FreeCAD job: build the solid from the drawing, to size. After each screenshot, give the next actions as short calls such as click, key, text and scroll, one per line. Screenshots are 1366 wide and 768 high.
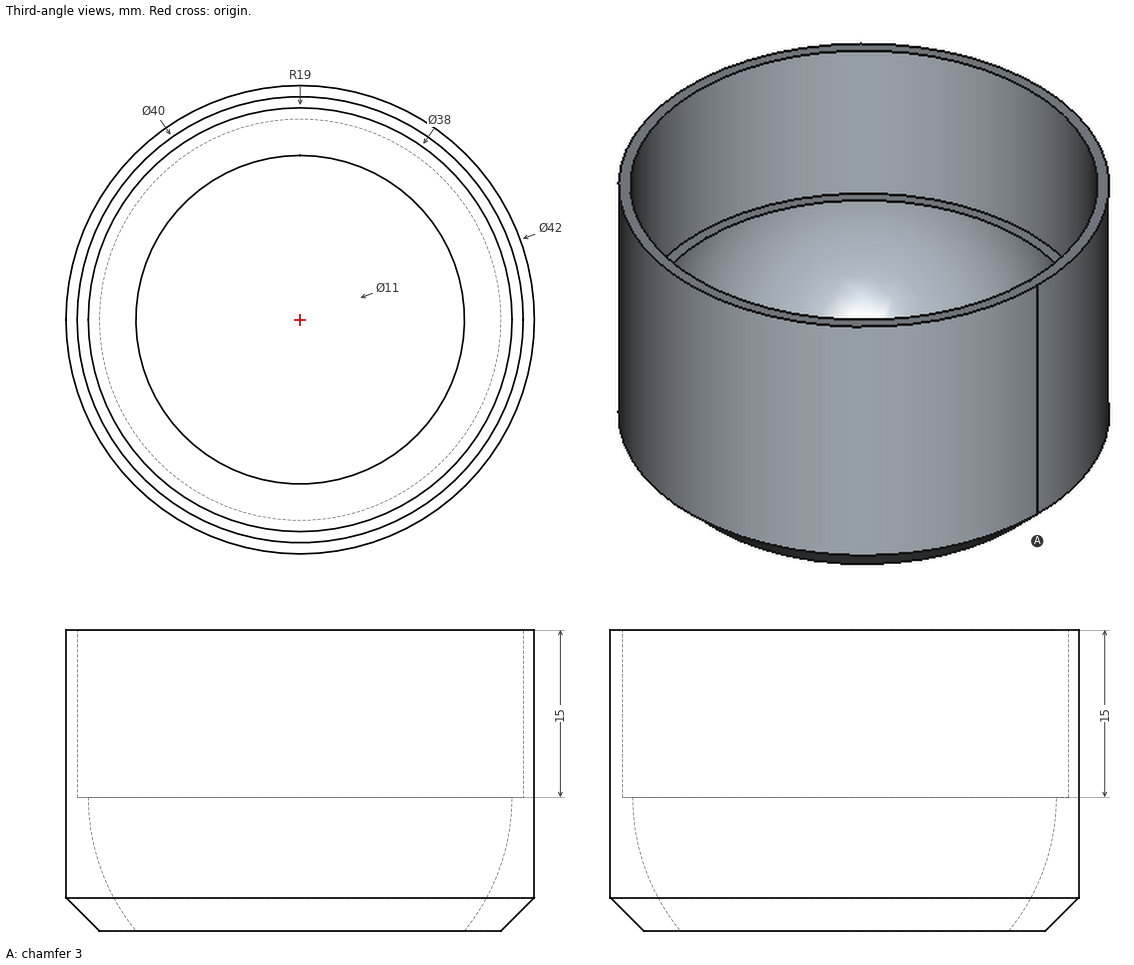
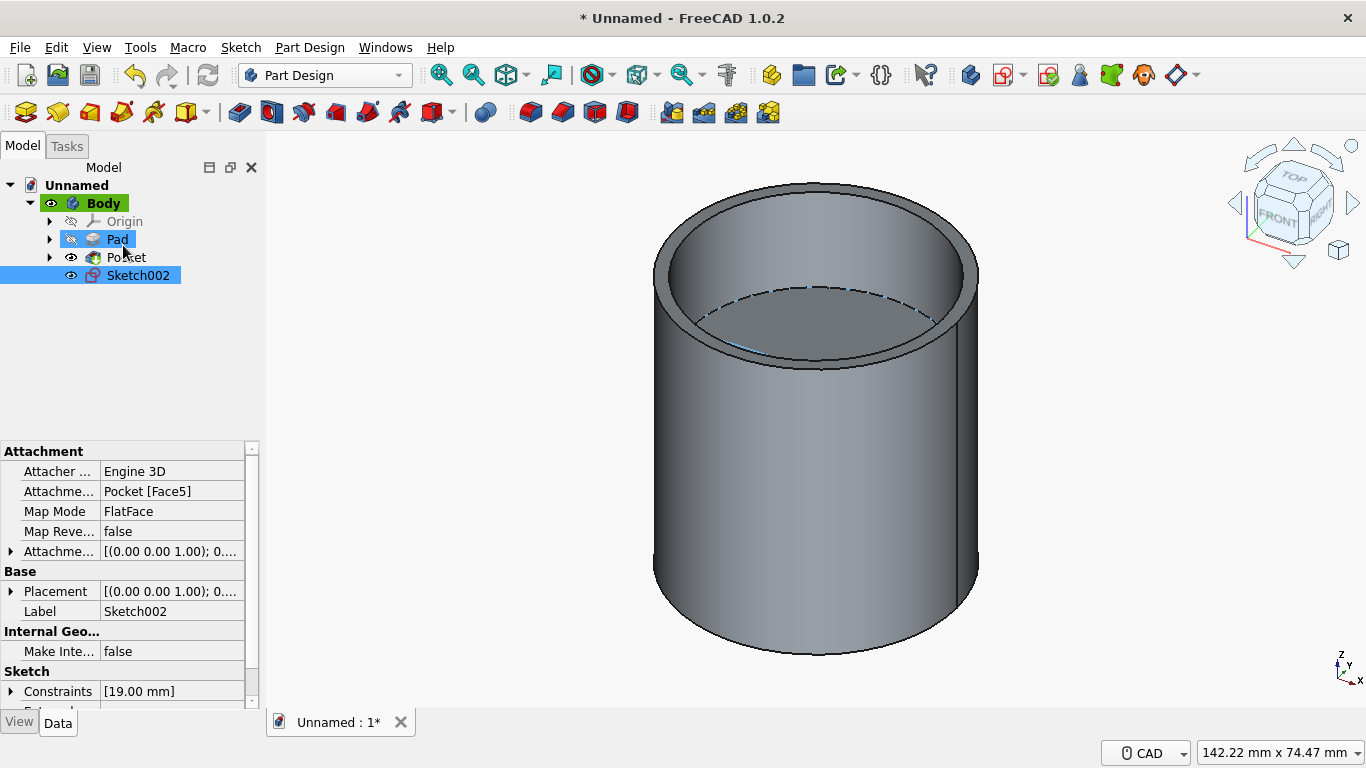
click(304, 112)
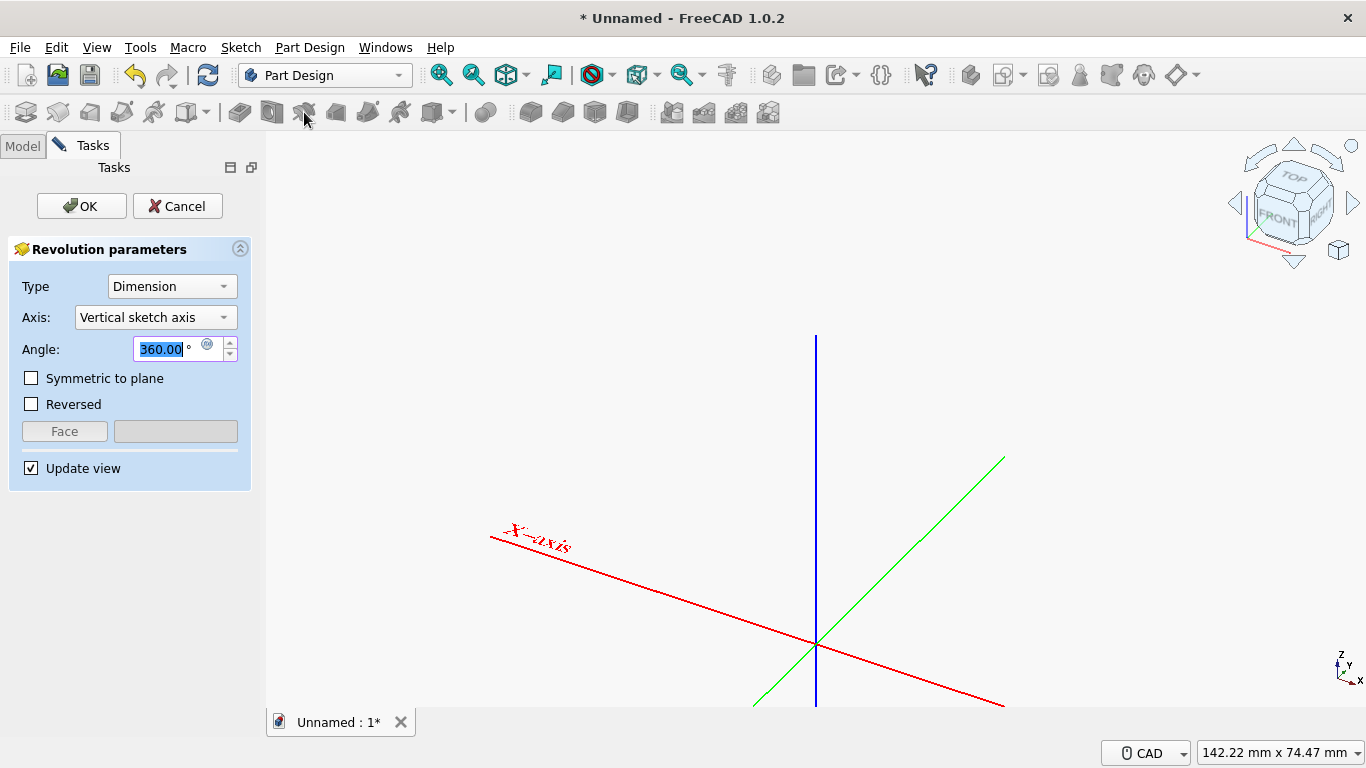
click(156, 318)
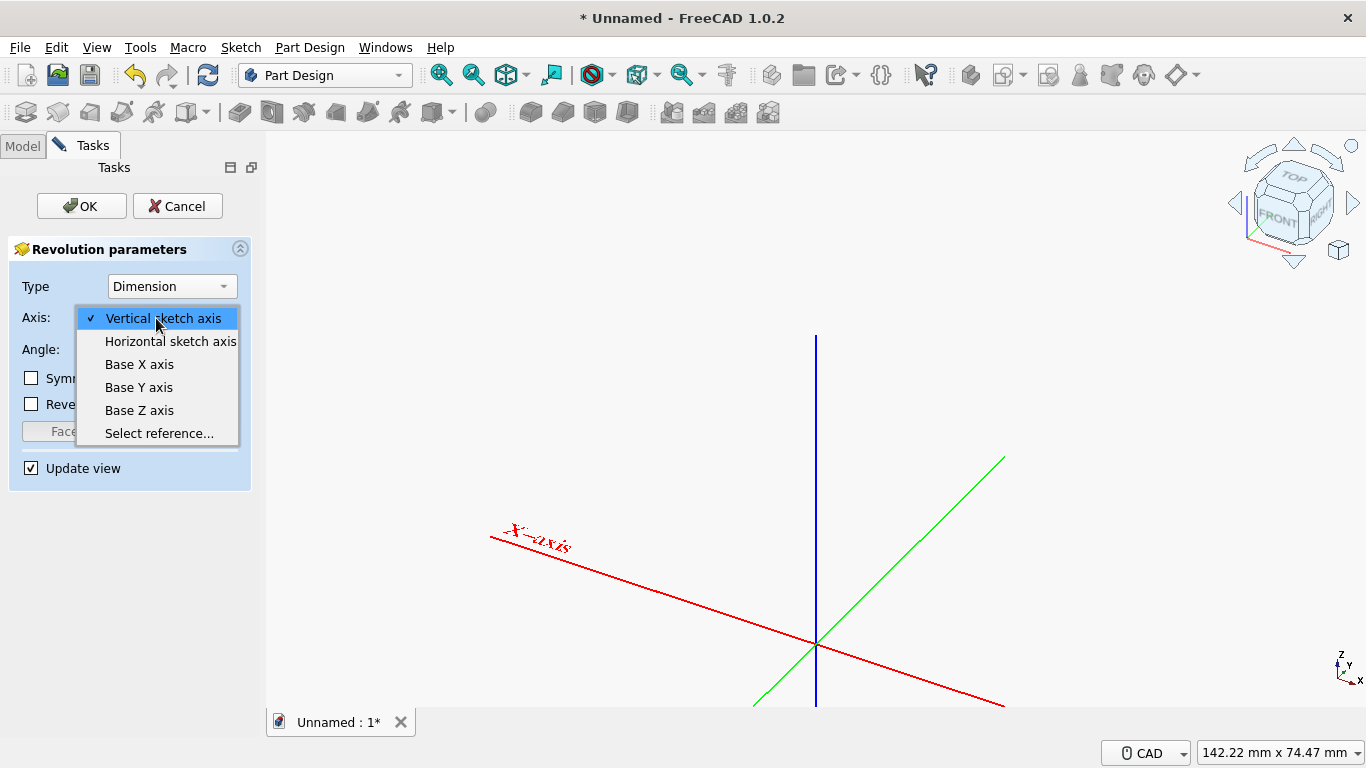
click(156, 342)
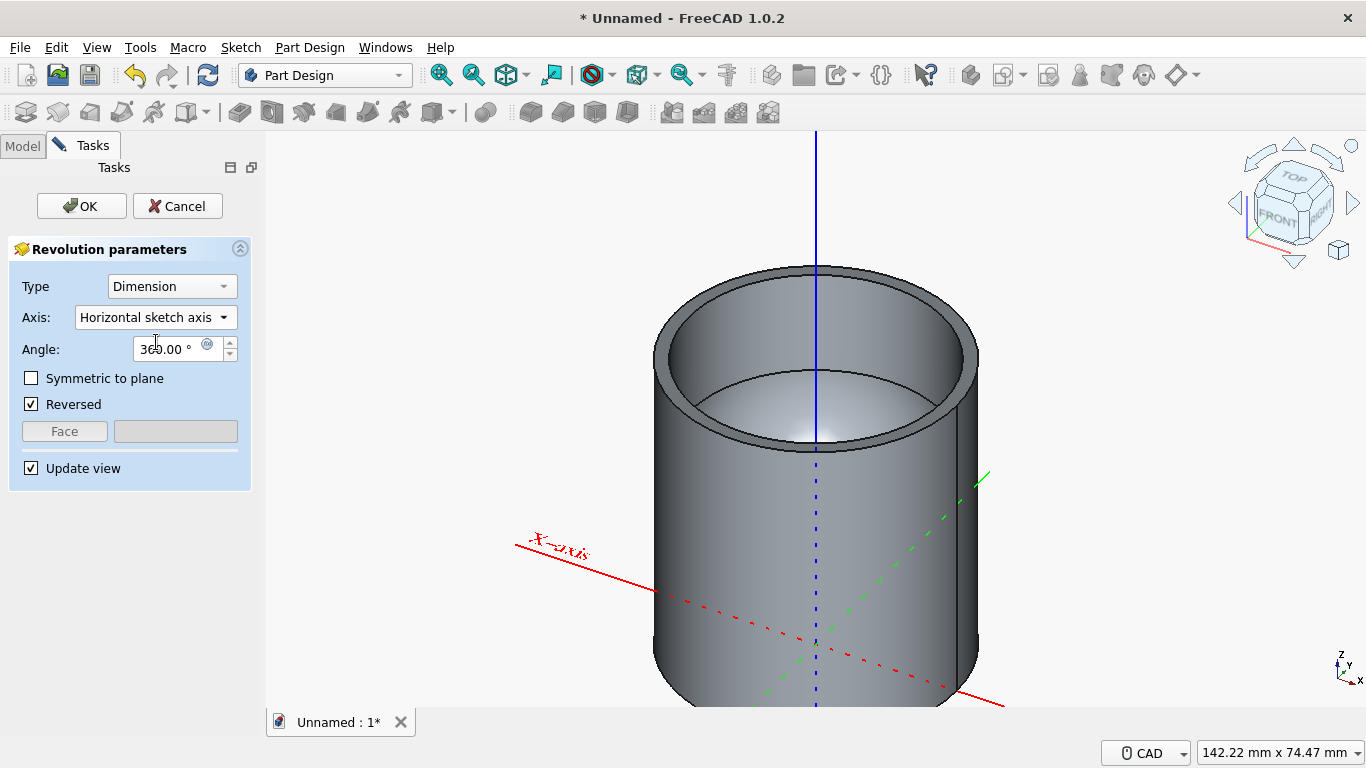
click(82, 206)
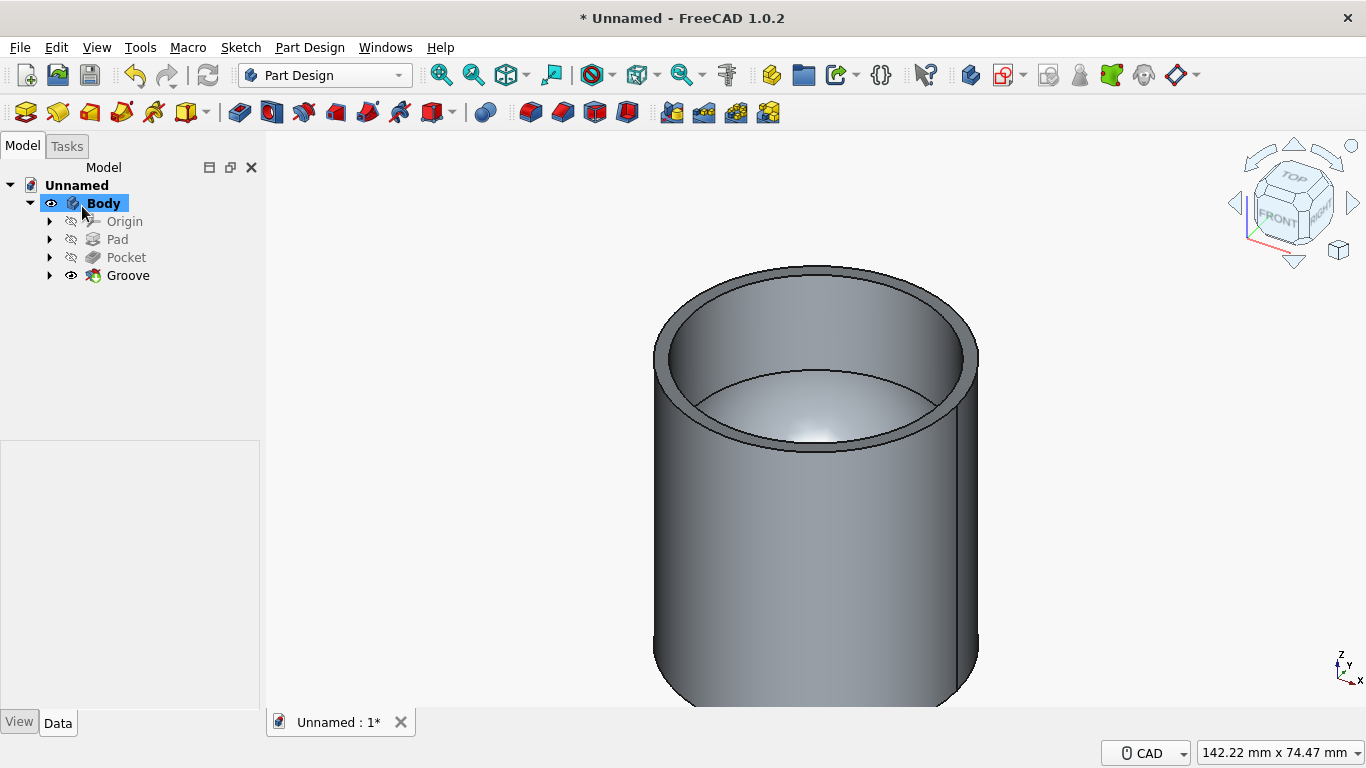
click(442, 76)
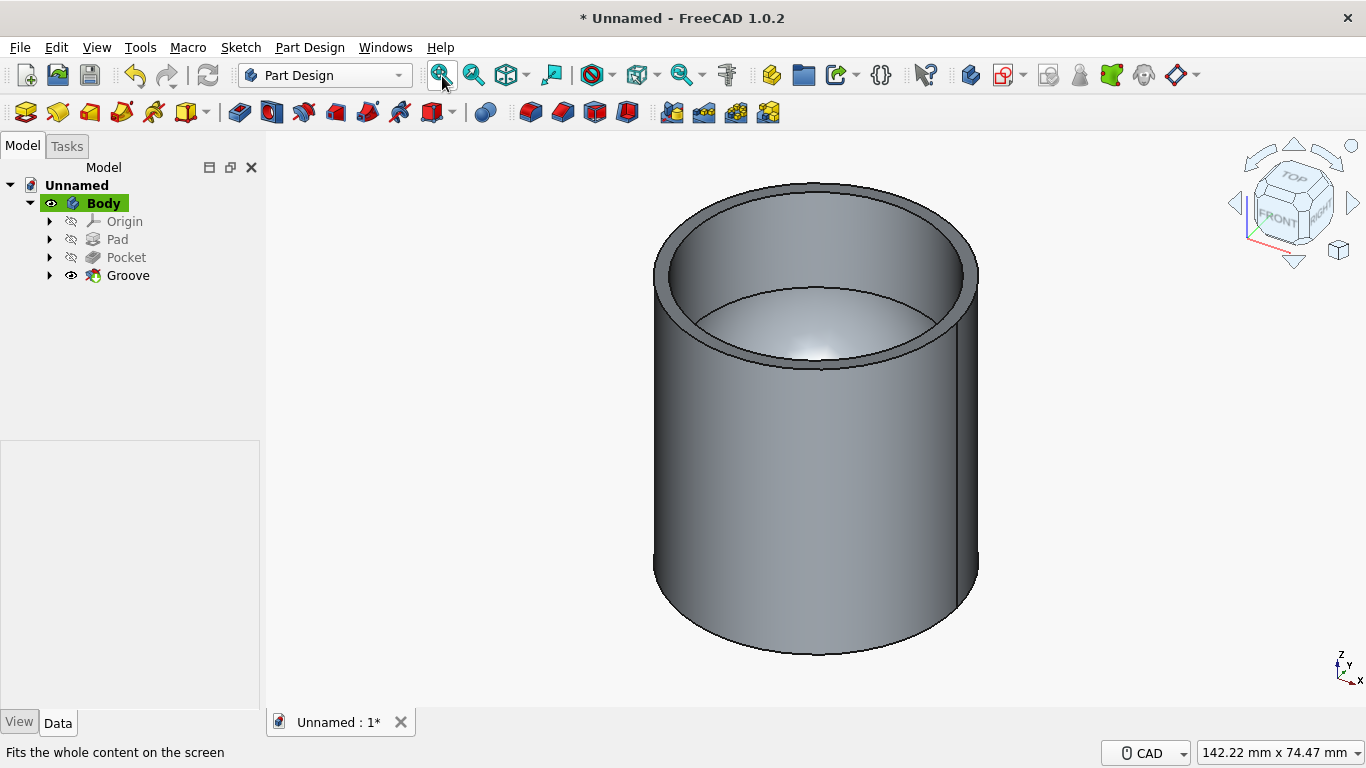
scroll(970, 294, up, 5)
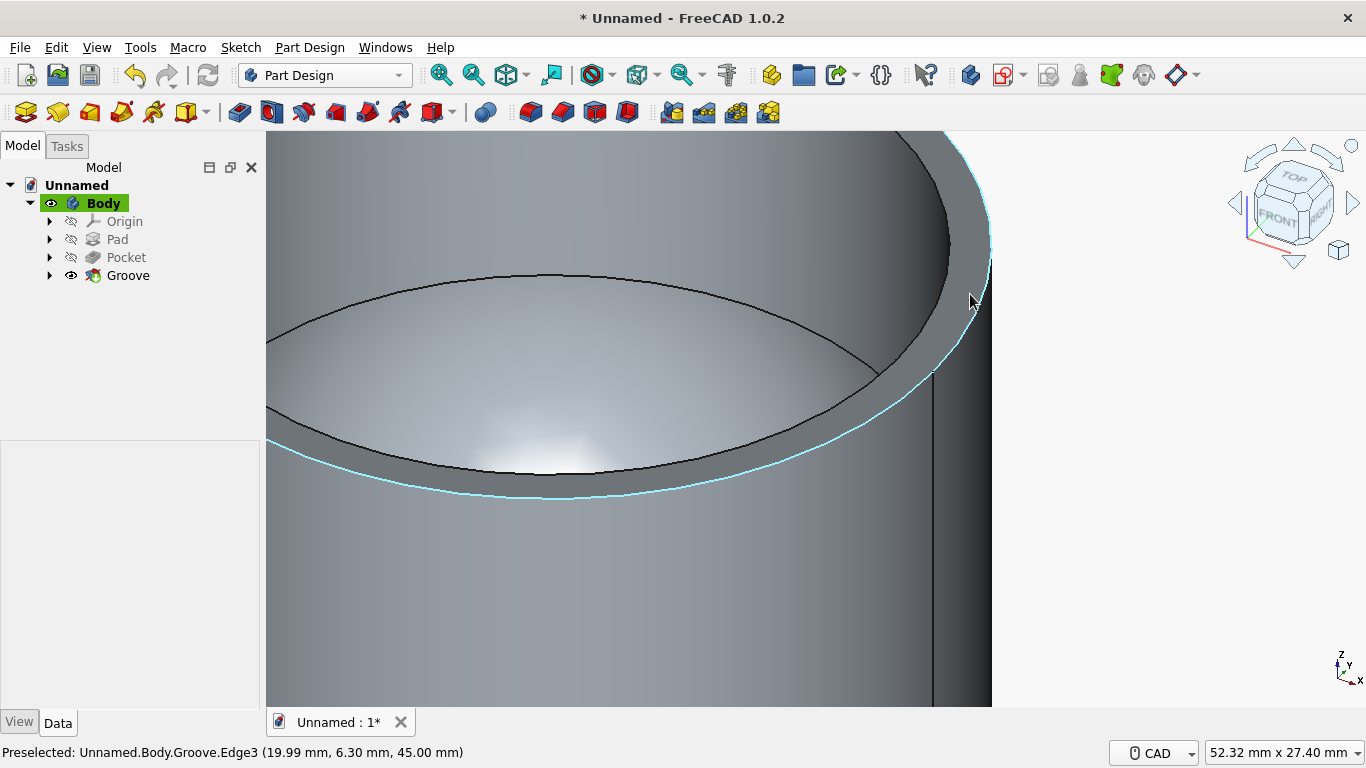
click(969, 295)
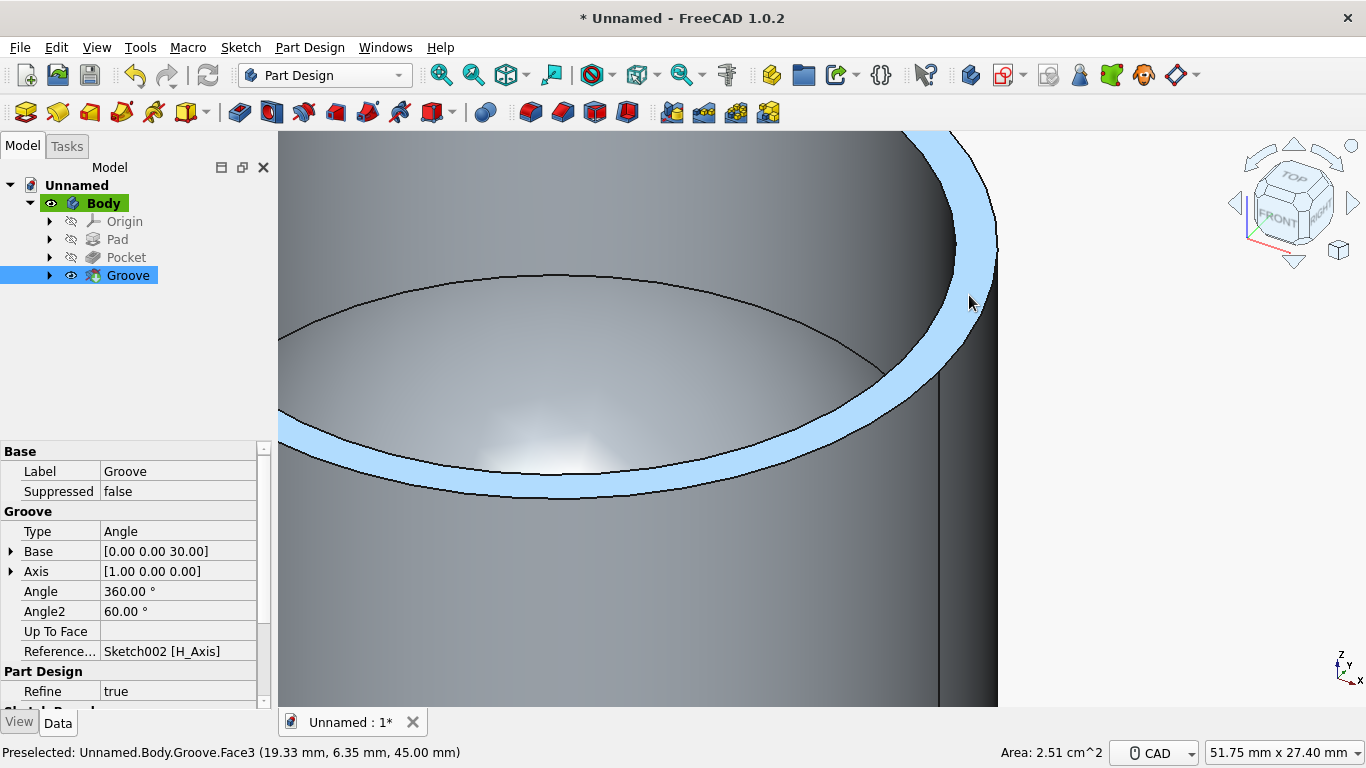
click(1004, 76)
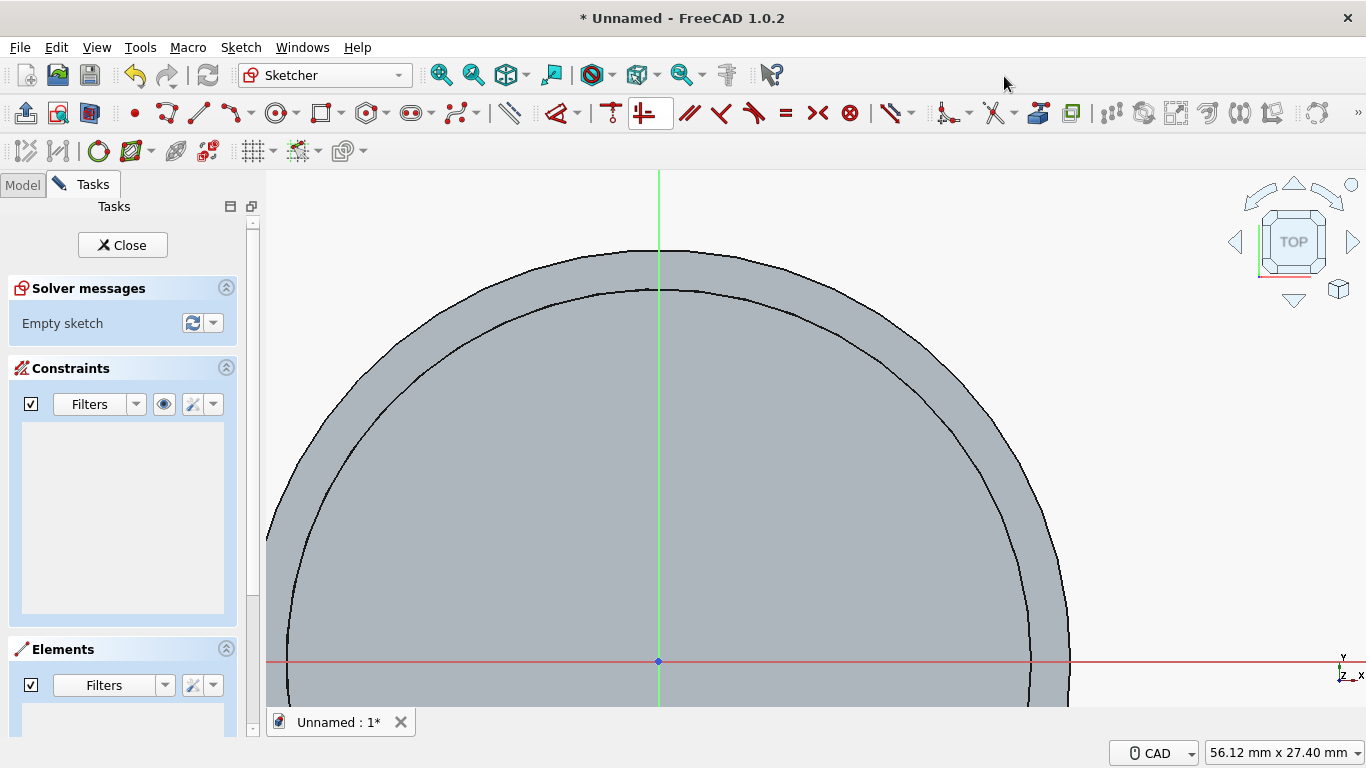
scroll(820, 256, down, 4)